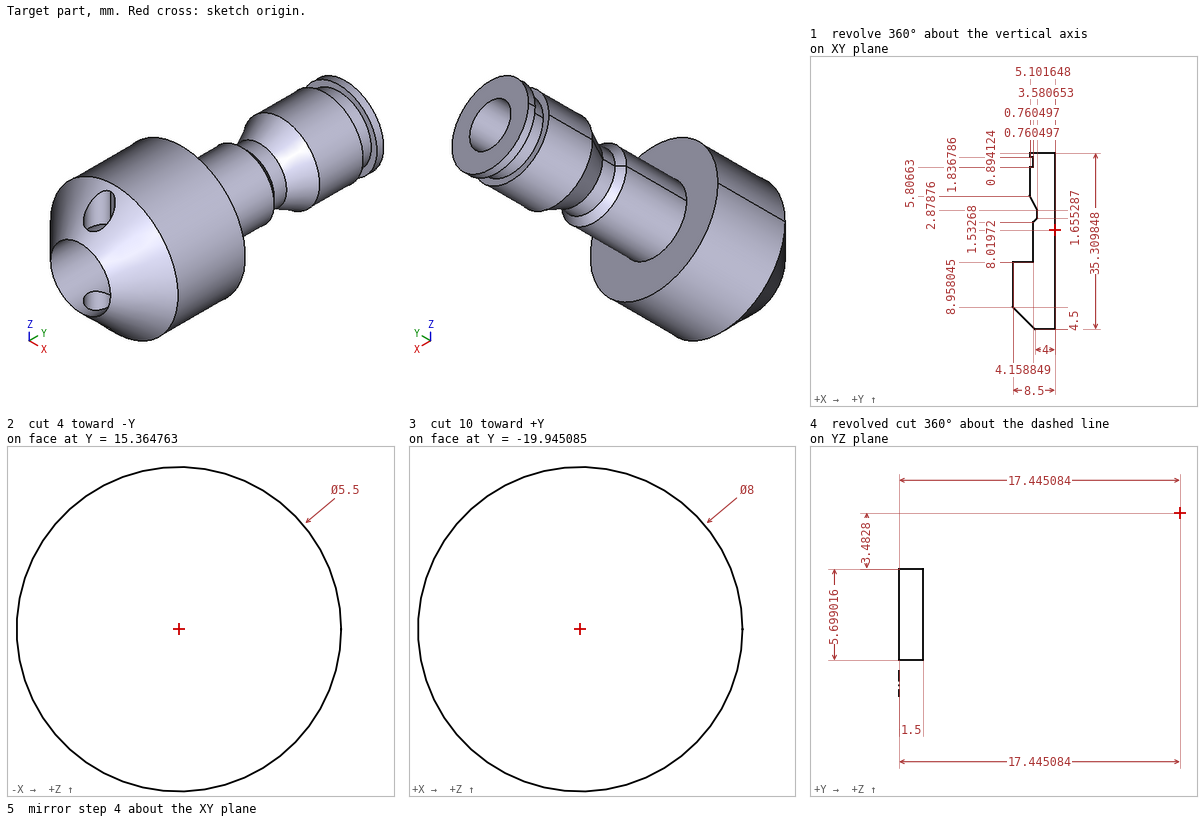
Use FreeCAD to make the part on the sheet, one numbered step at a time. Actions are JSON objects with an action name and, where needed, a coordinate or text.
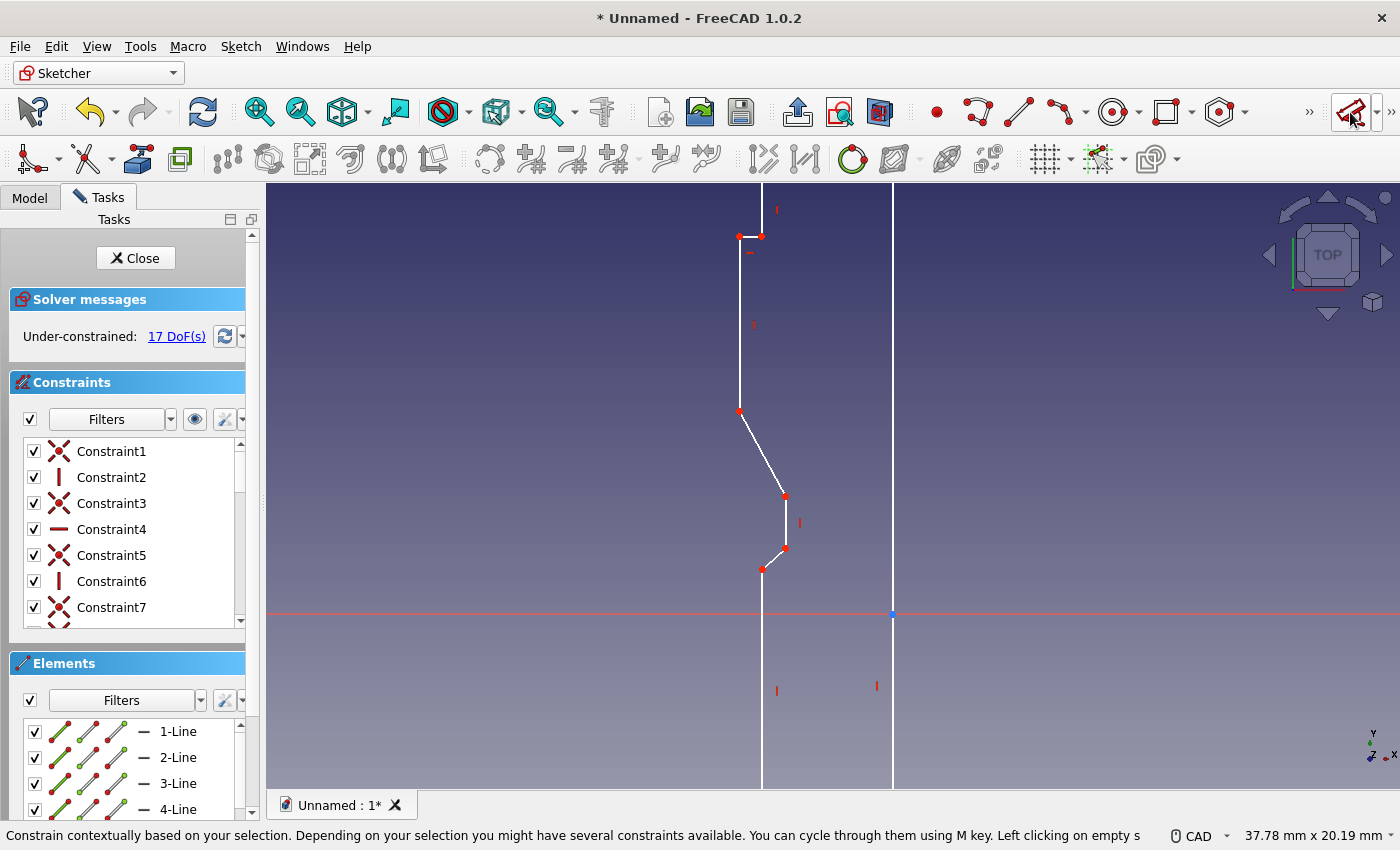
{"action": "scroll", "coordinate": [764, 371], "scroll_direction": "down", "scroll_amount": 5}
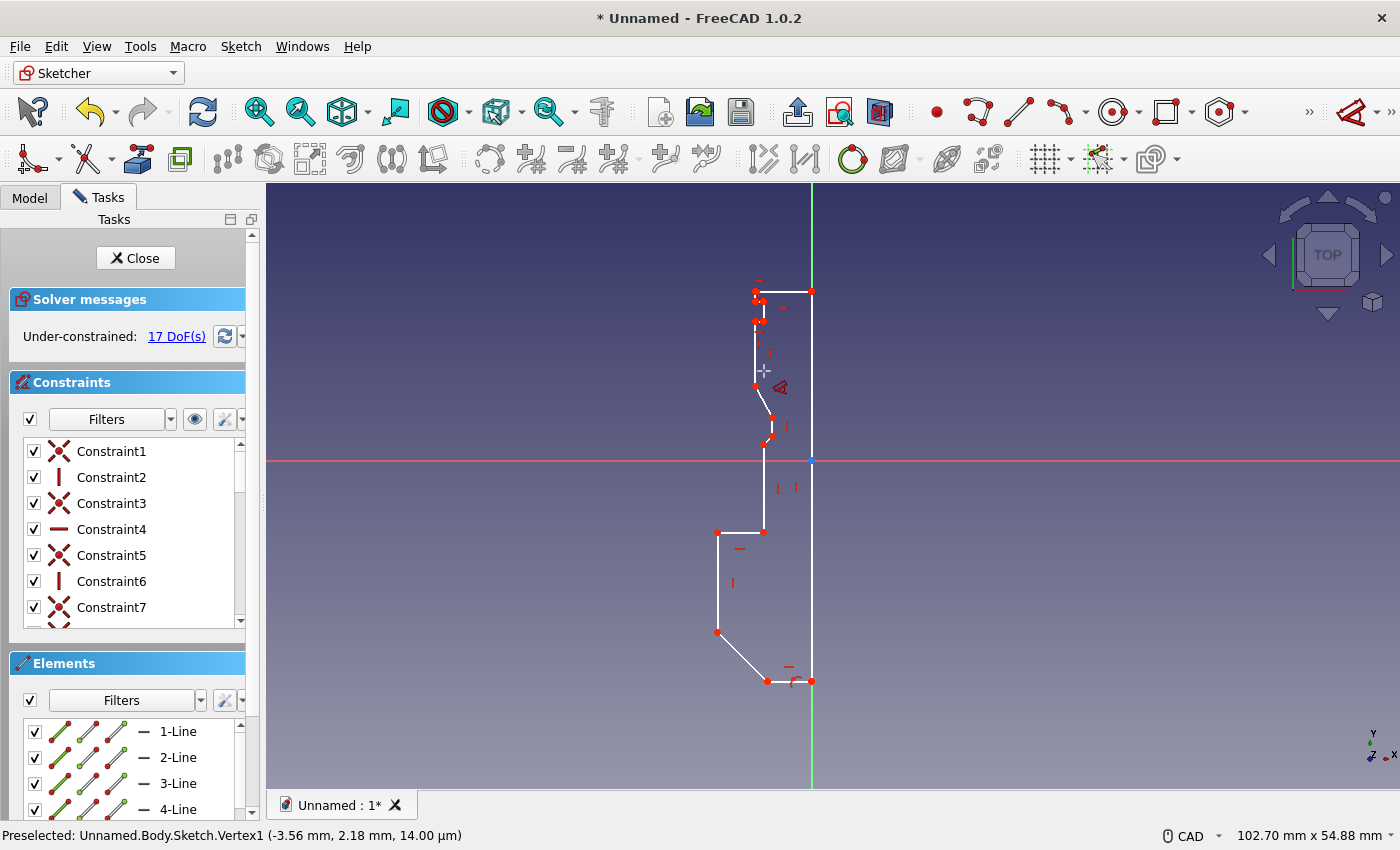
{"action": "left_click", "coordinate": [780, 682]}
{"action": "left_click", "coordinate": [789, 716]}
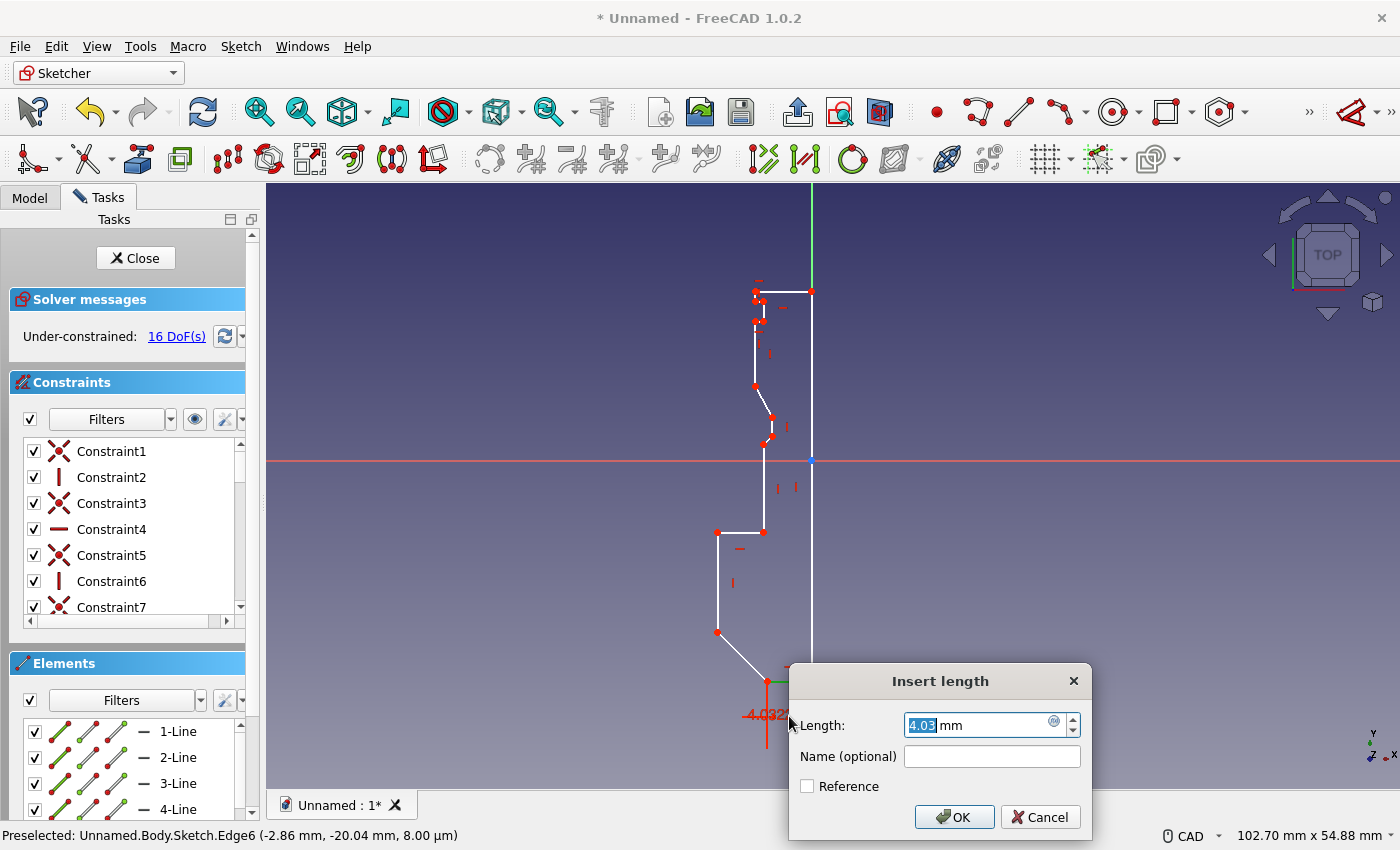
{"action": "type", "text": "4"}
{"action": "key", "text": "Return"}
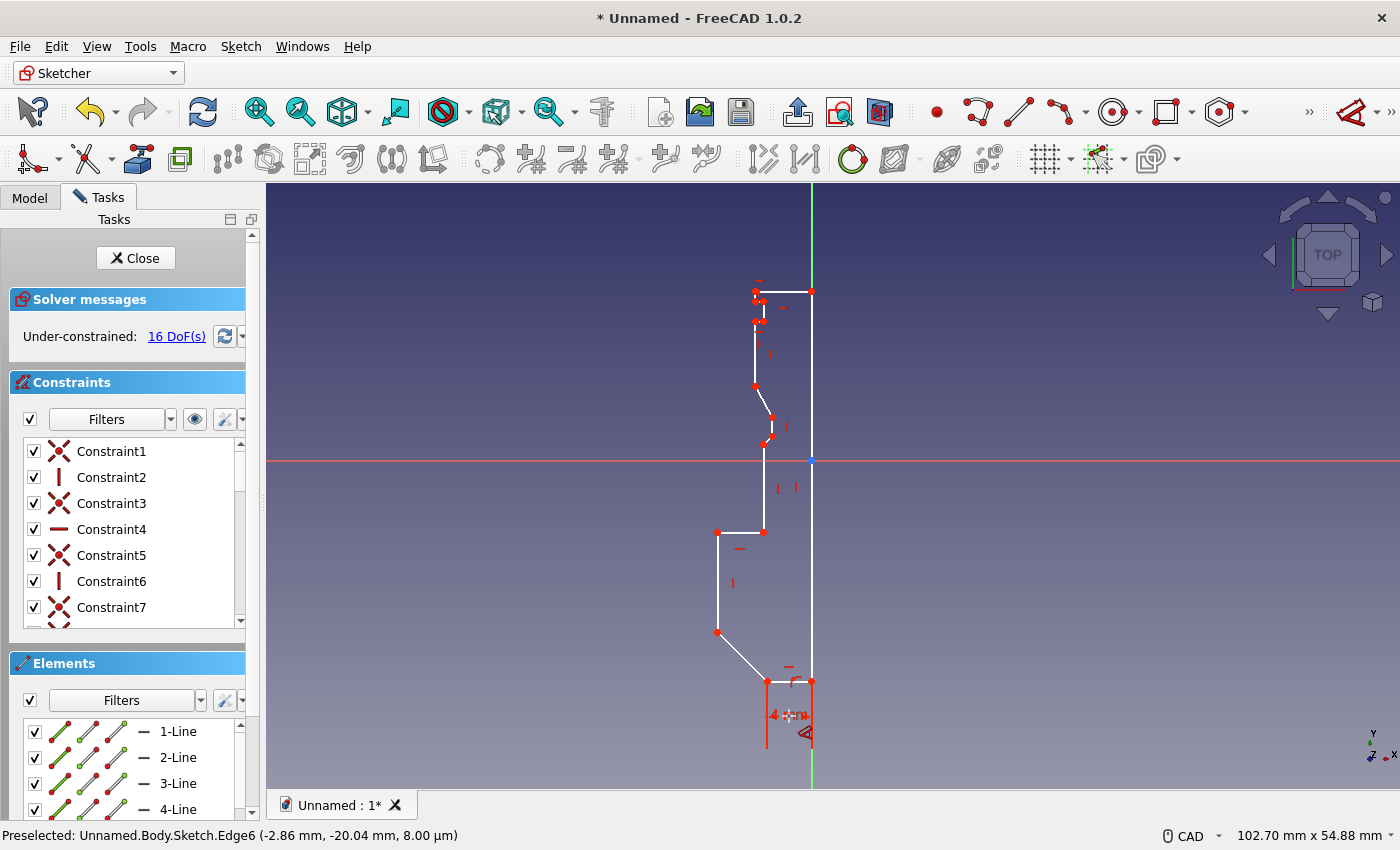
{"action": "left_click", "coordinate": [718, 533]}
{"action": "left_click", "coordinate": [765, 567]}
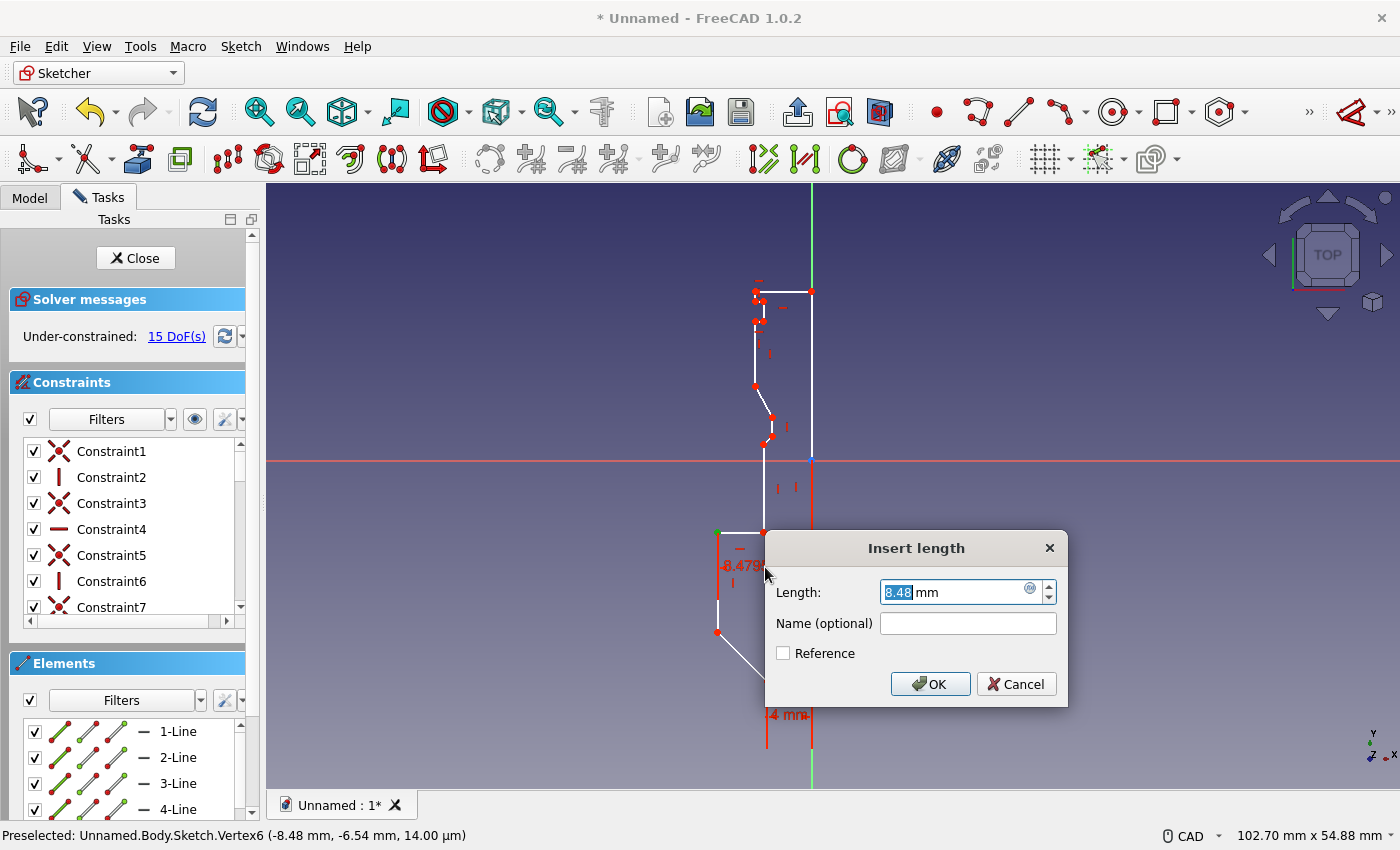
{"action": "type", "text": "8.5"}
{"action": "key", "text": "Return"}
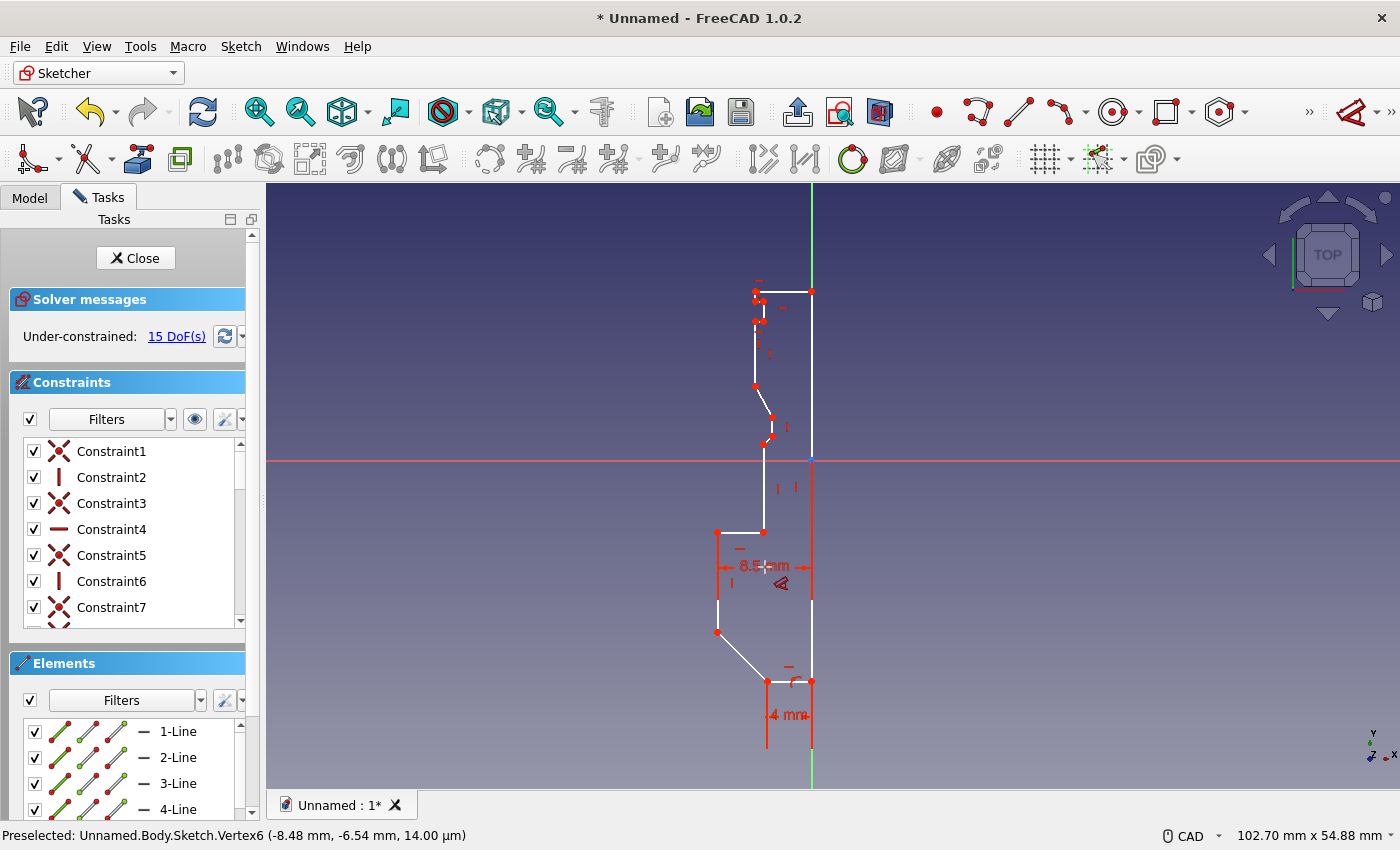
{"action": "left_click", "coordinate": [733, 647]}
{"action": "left_click", "coordinate": [684, 657]}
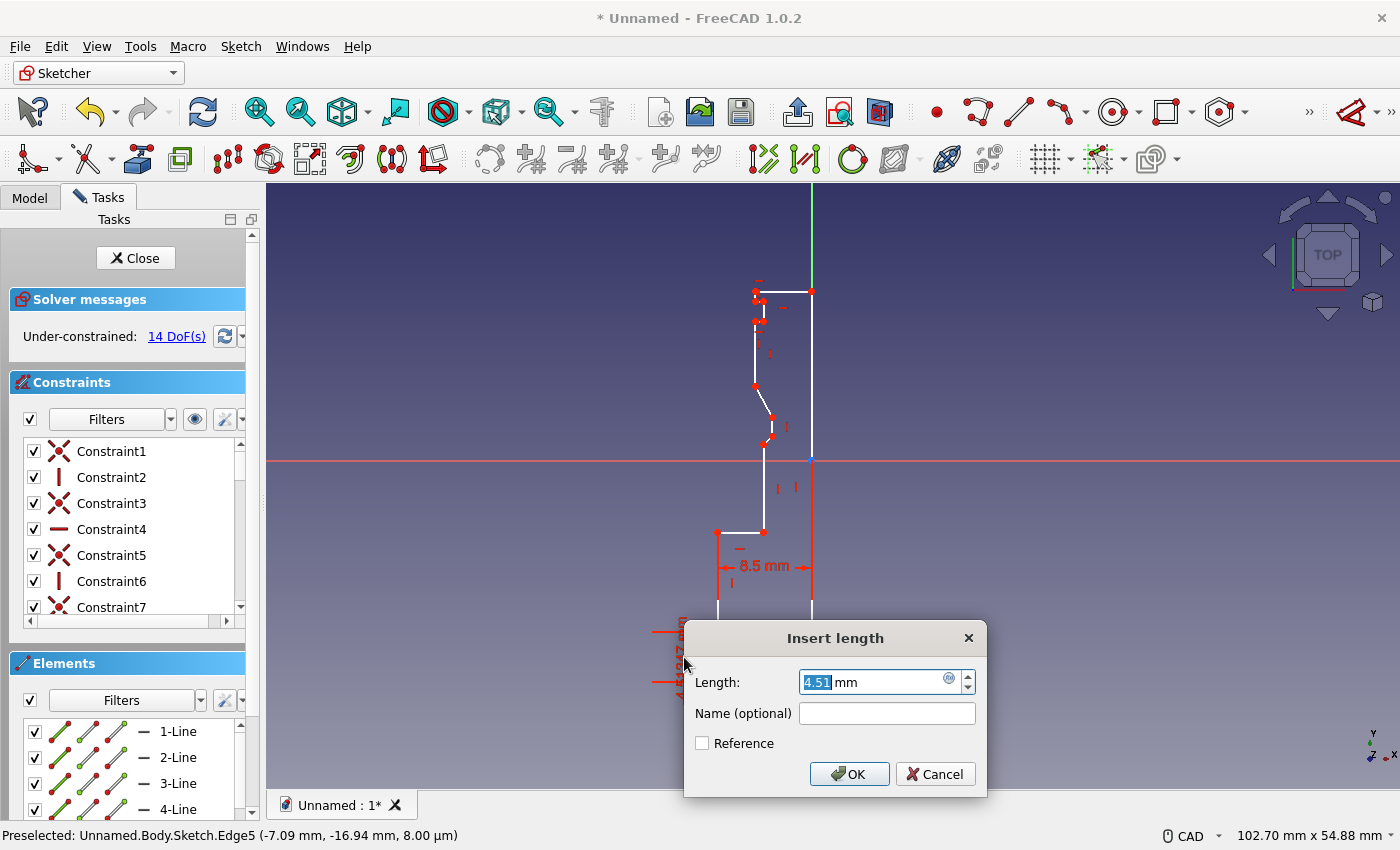
{"action": "type", "text": "4.5"}
{"action": "key", "text": "Return"}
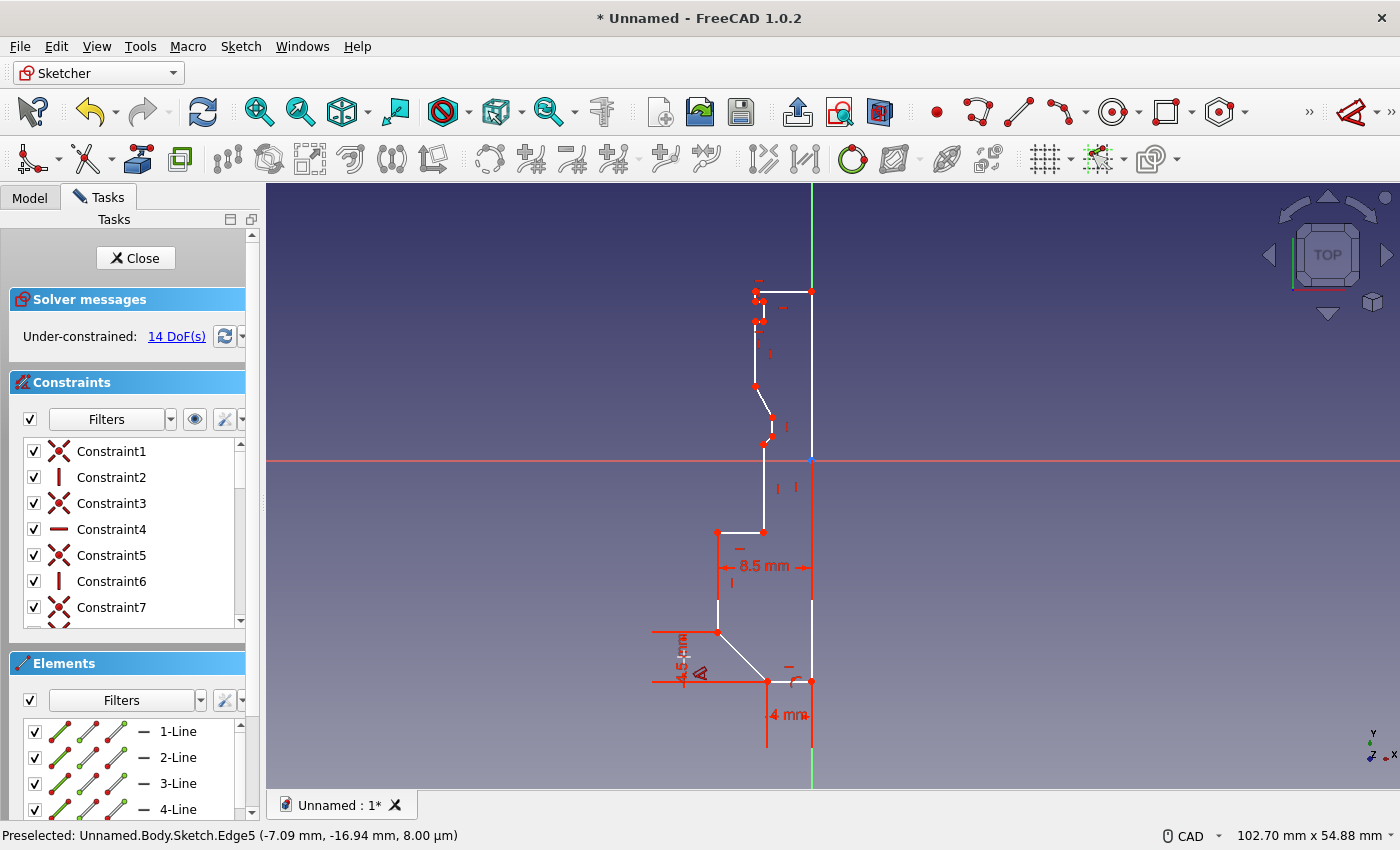
{"action": "scroll", "coordinate": [764, 471], "scroll_direction": "up", "scroll_amount": 2}